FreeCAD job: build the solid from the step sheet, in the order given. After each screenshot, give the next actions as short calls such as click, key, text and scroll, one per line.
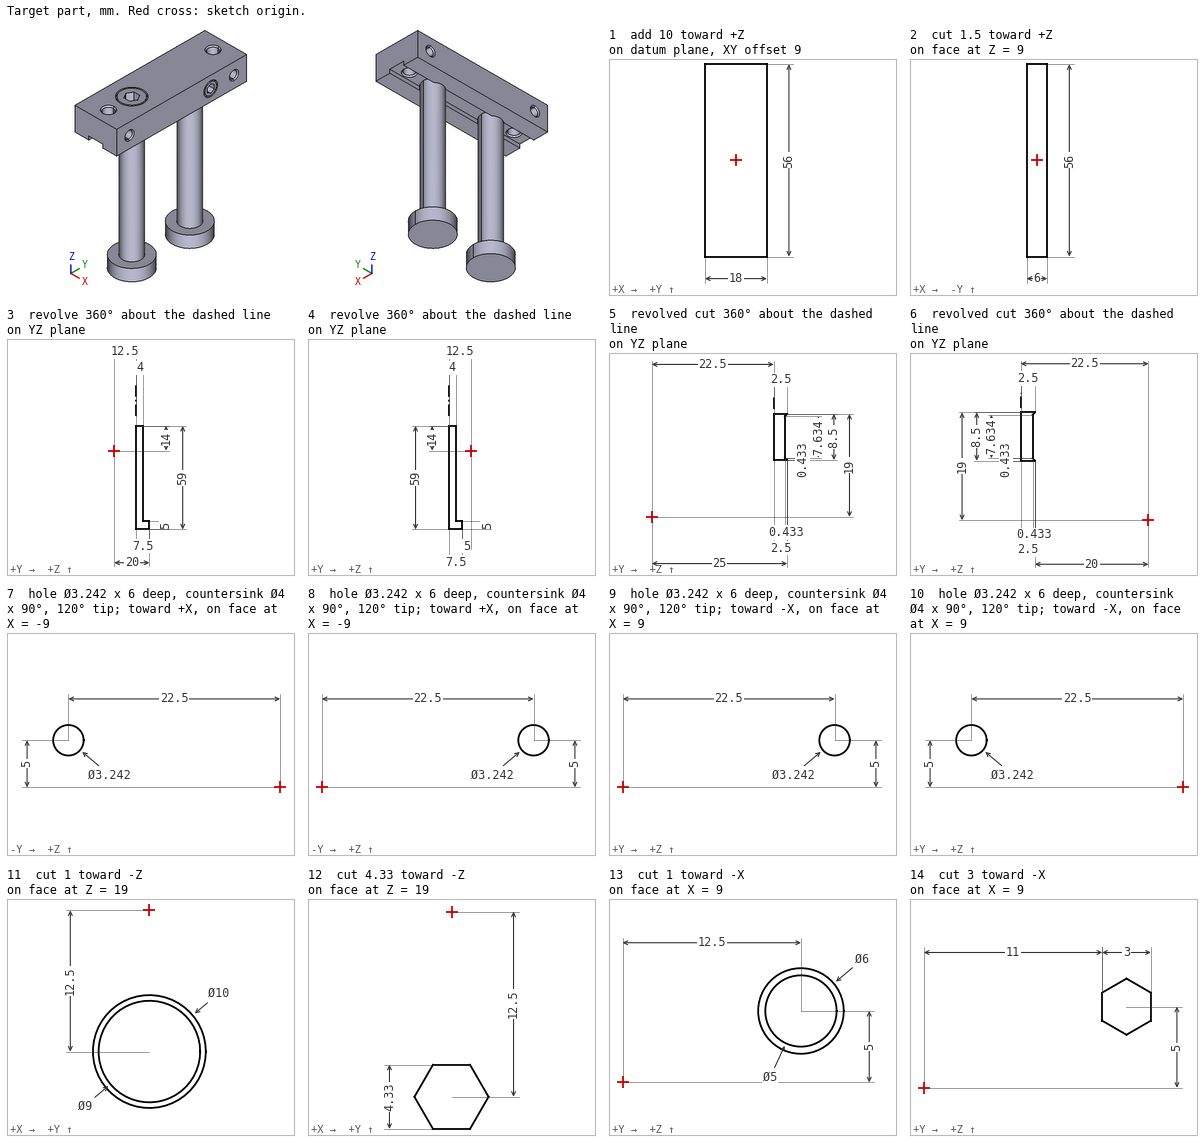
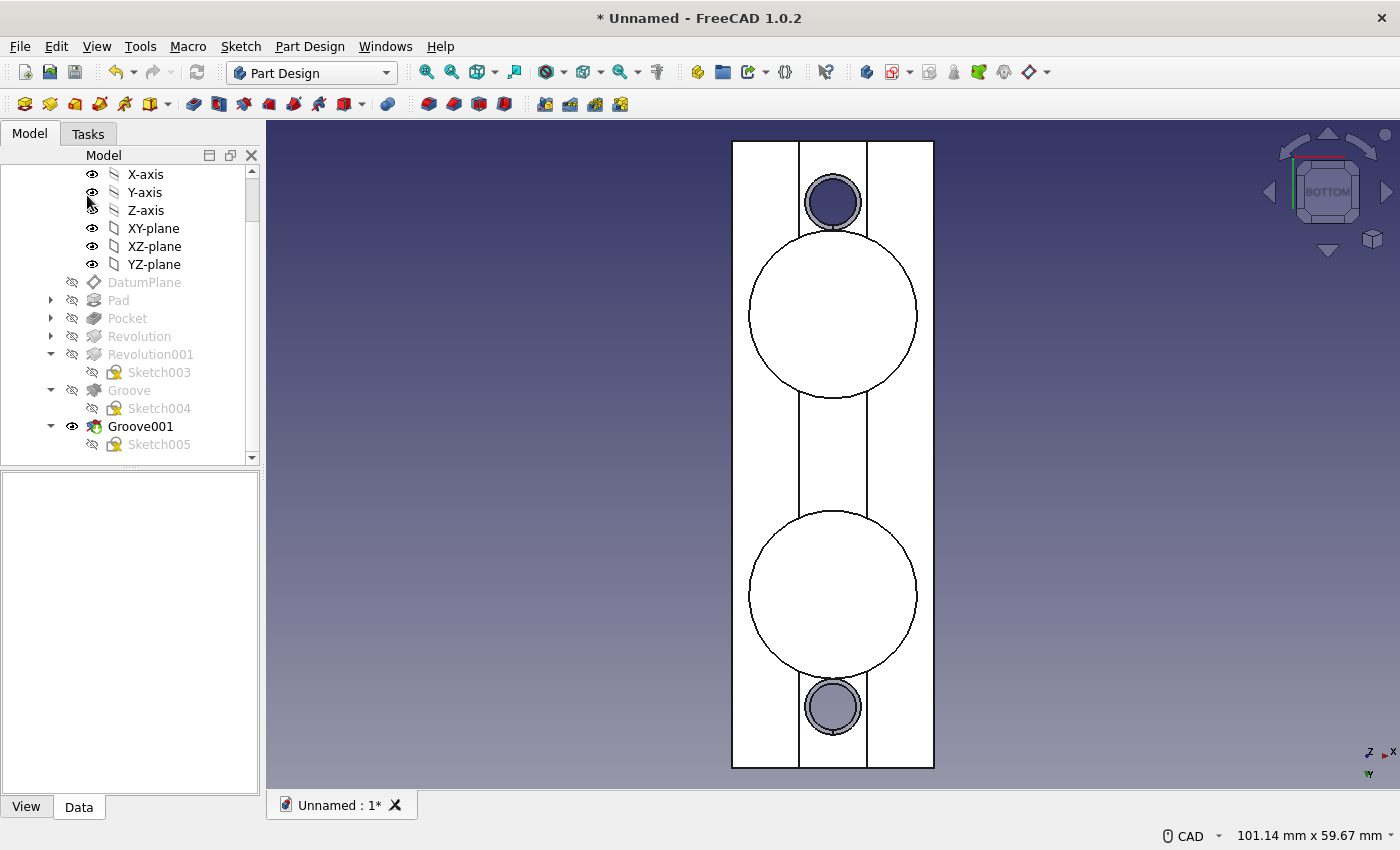
key(6)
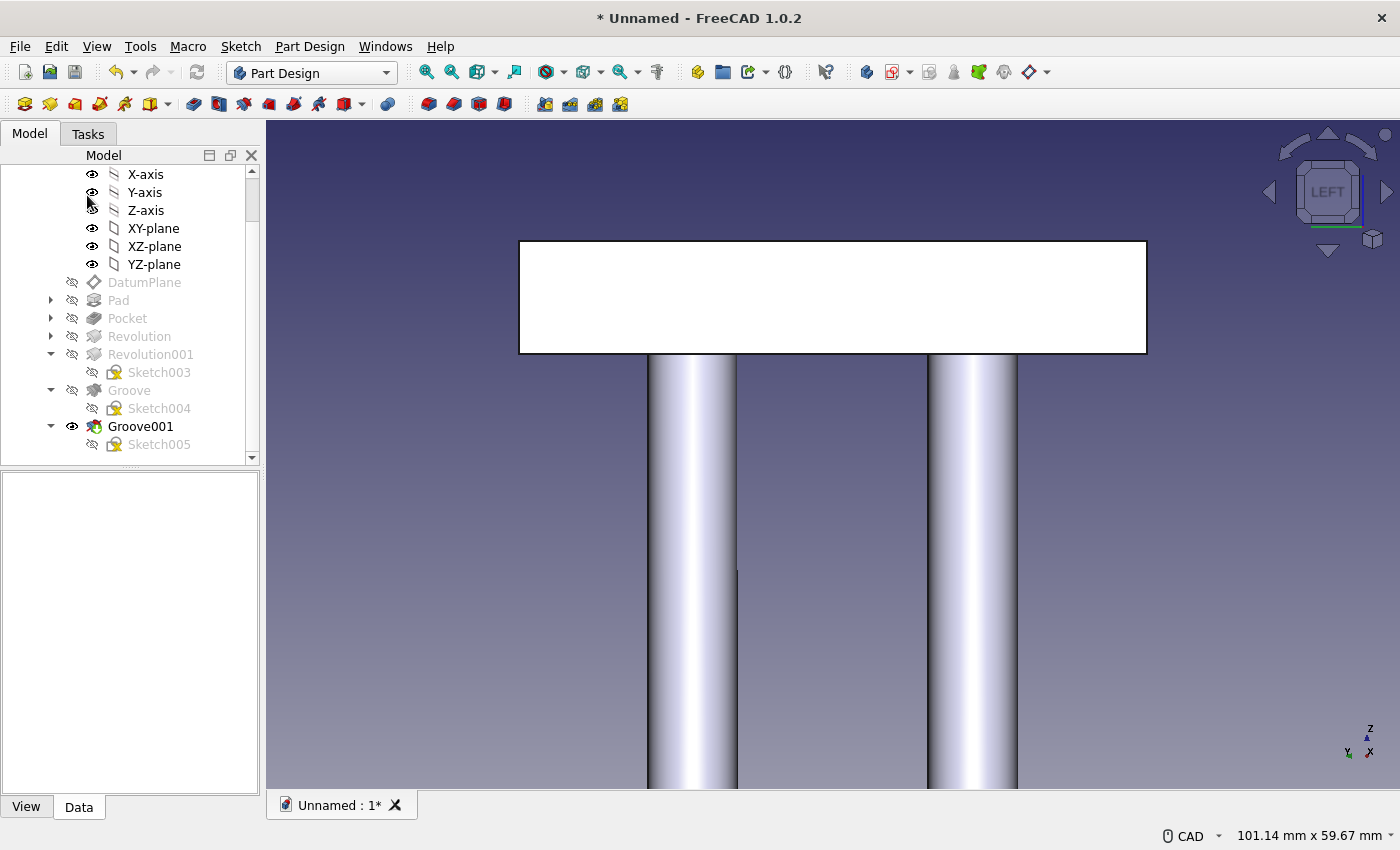
click(427, 72)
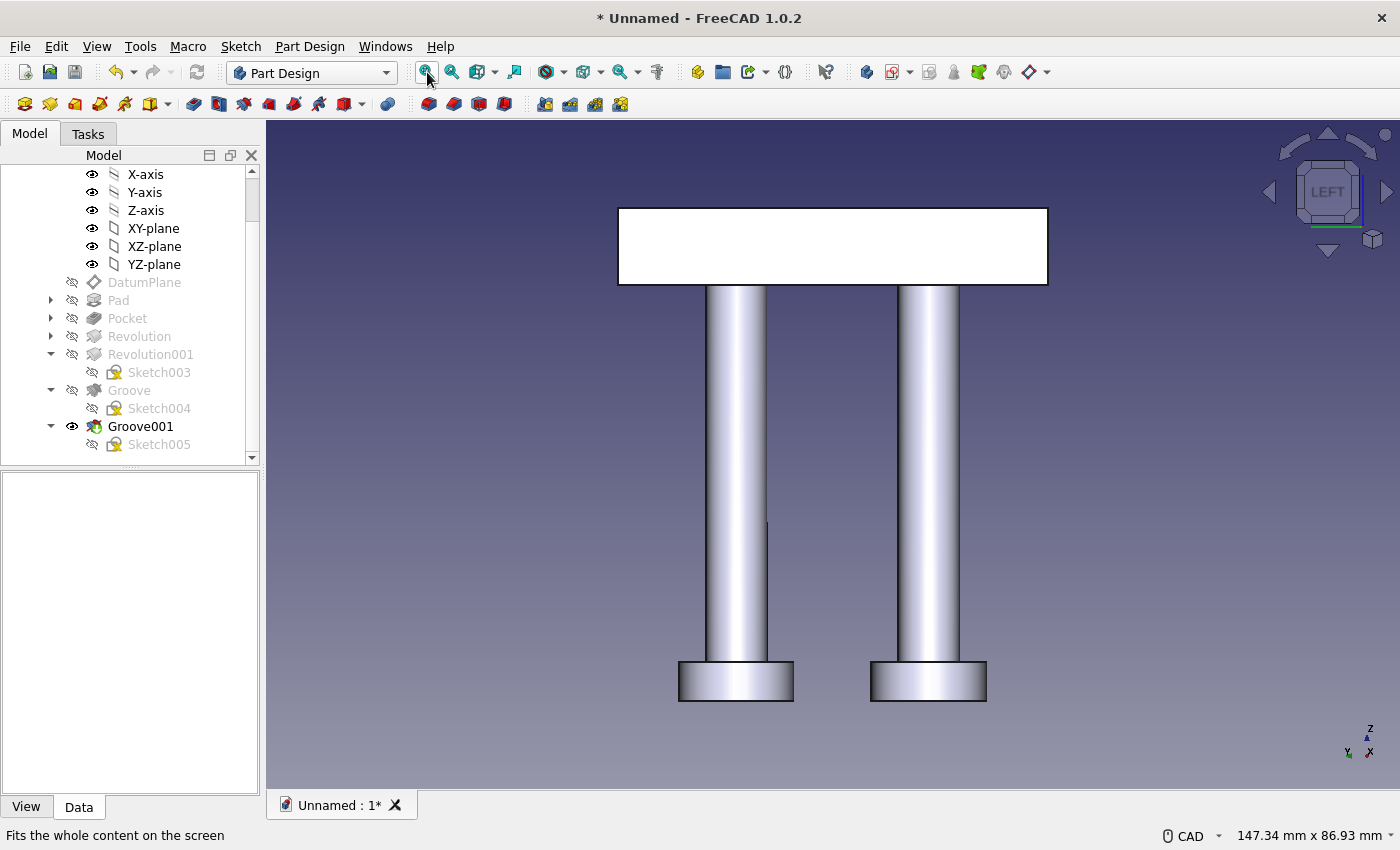
click(710, 246)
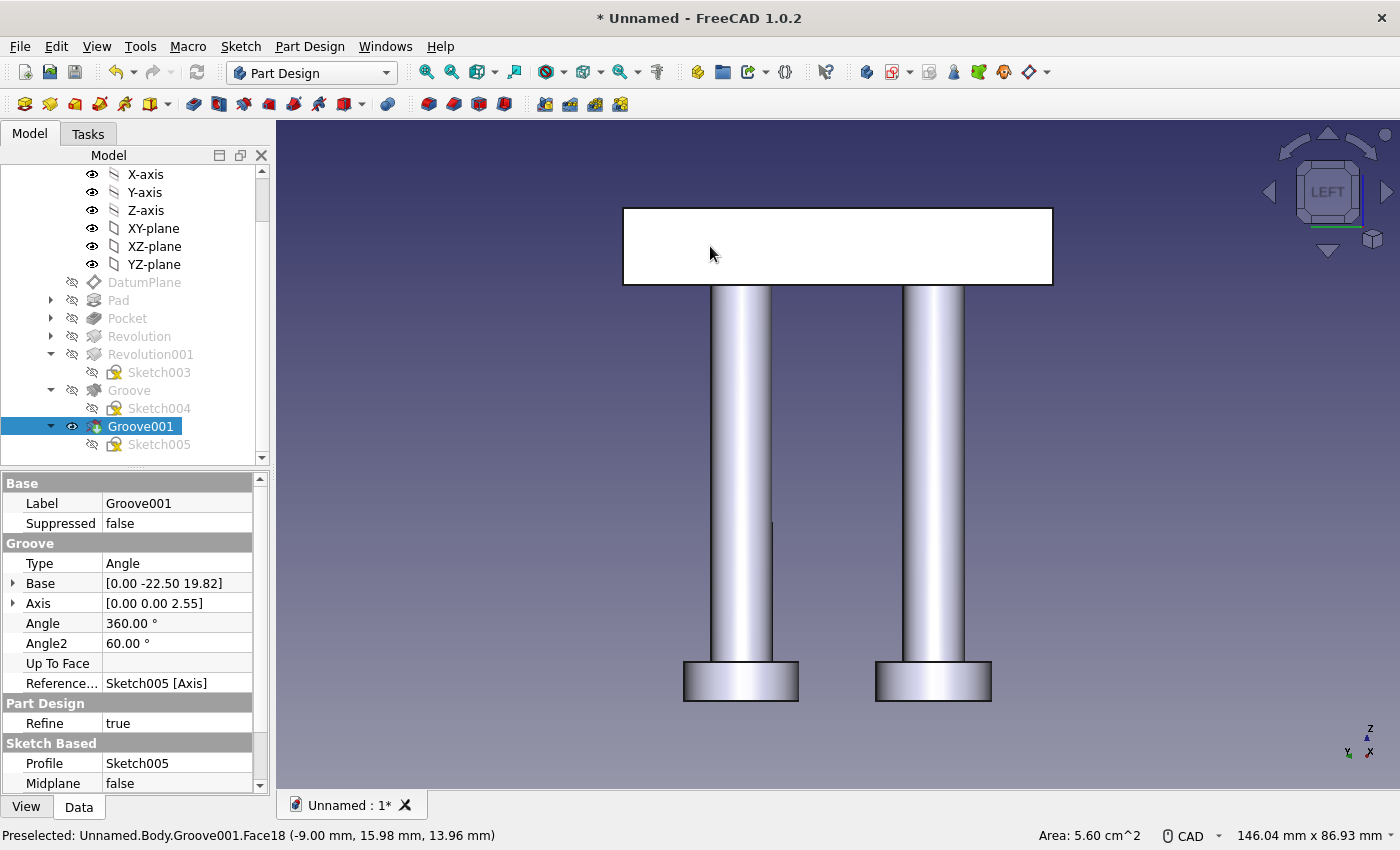
click(892, 72)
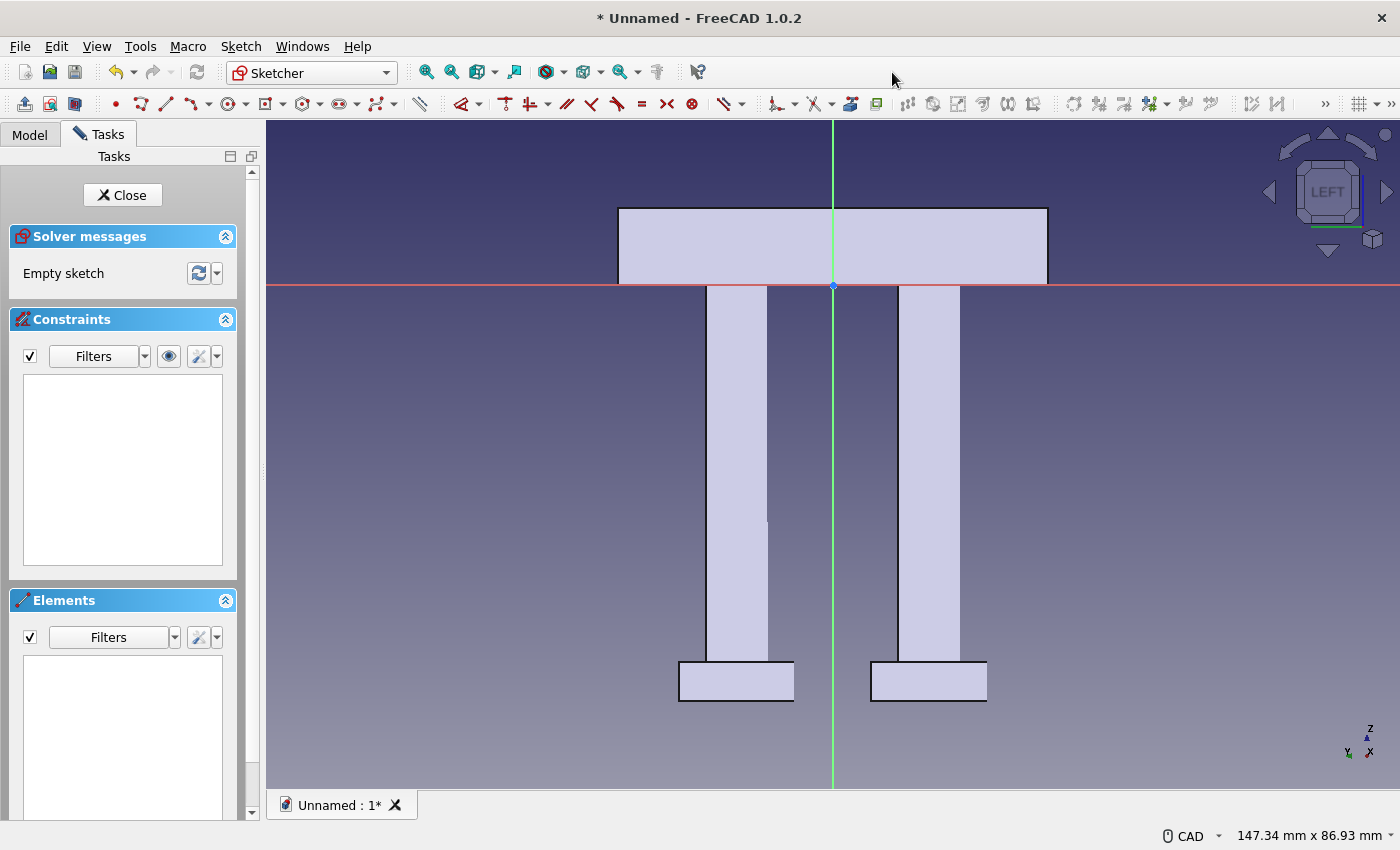
scroll(653, 233, up, 14)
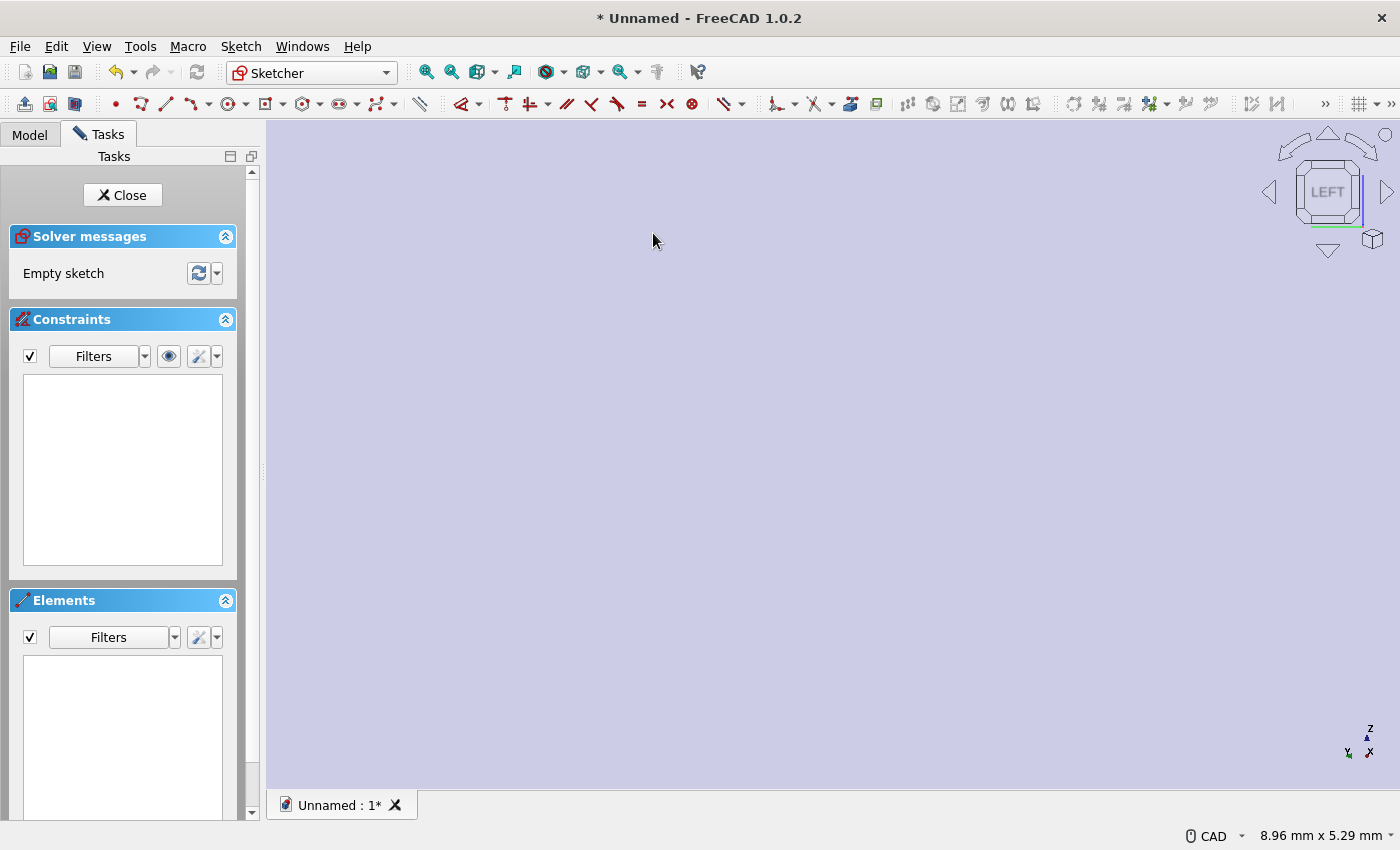
click(228, 104)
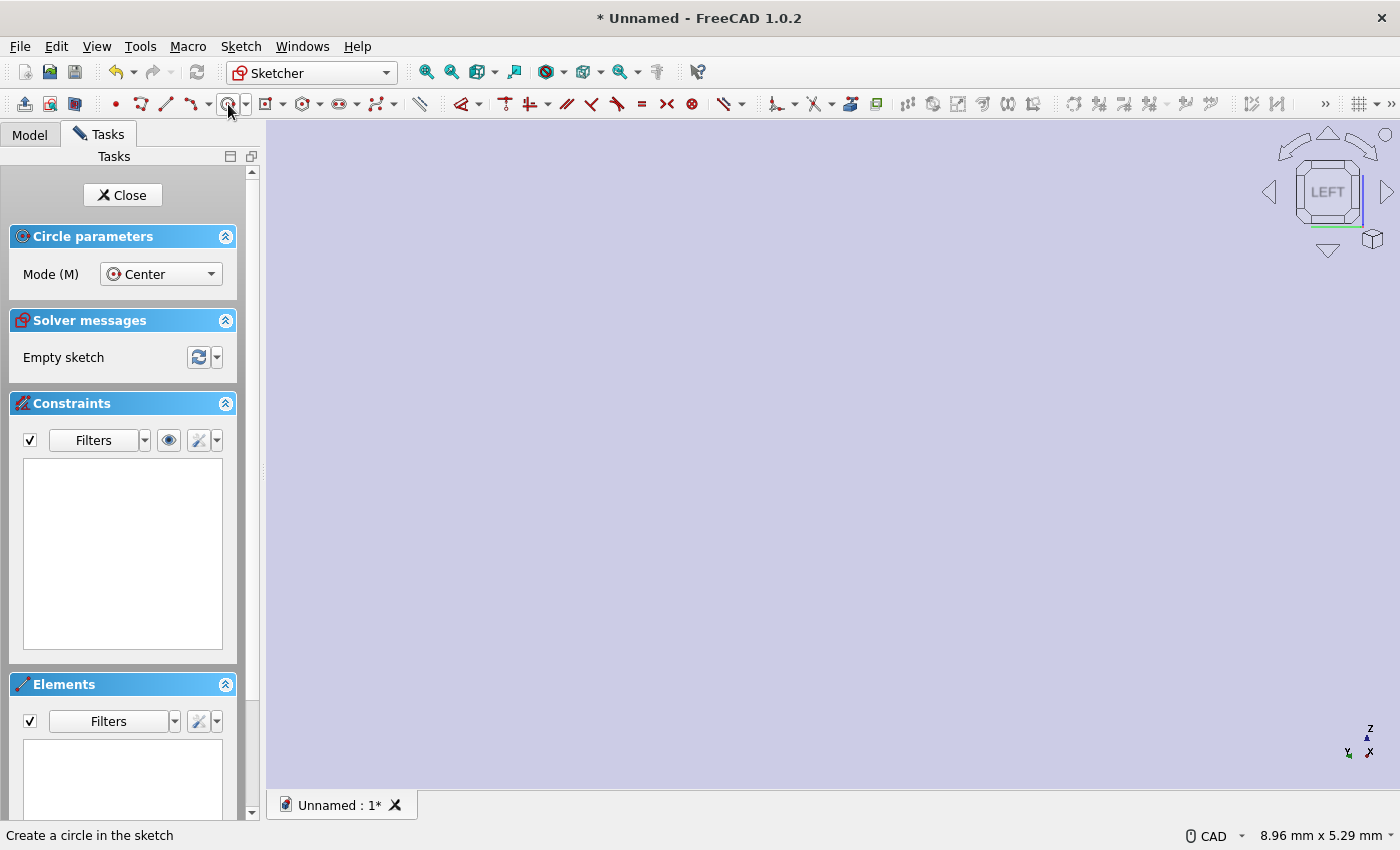
click(760, 456)
move(905, 311)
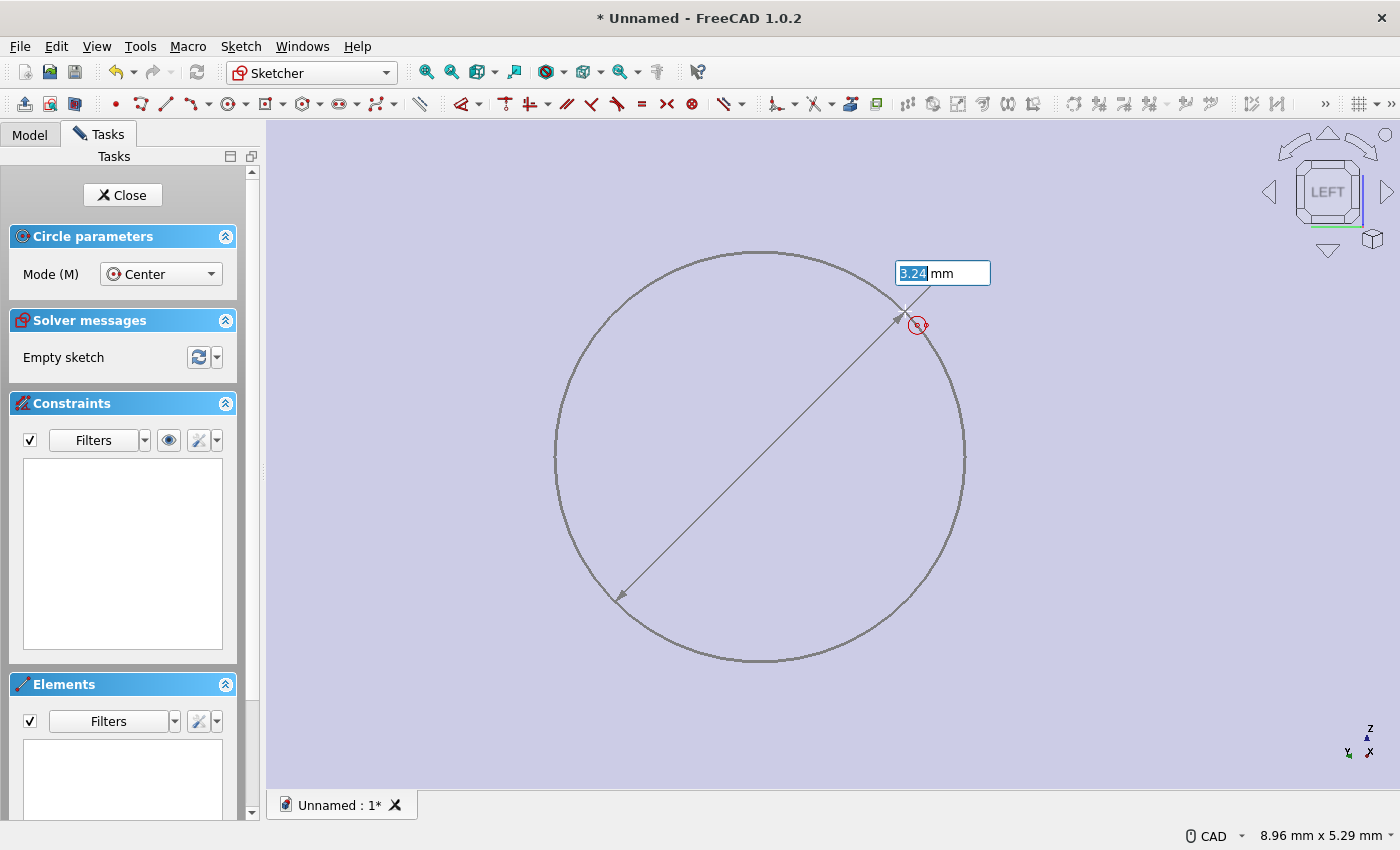
text(3.242)
key(Return)
key(Escape)